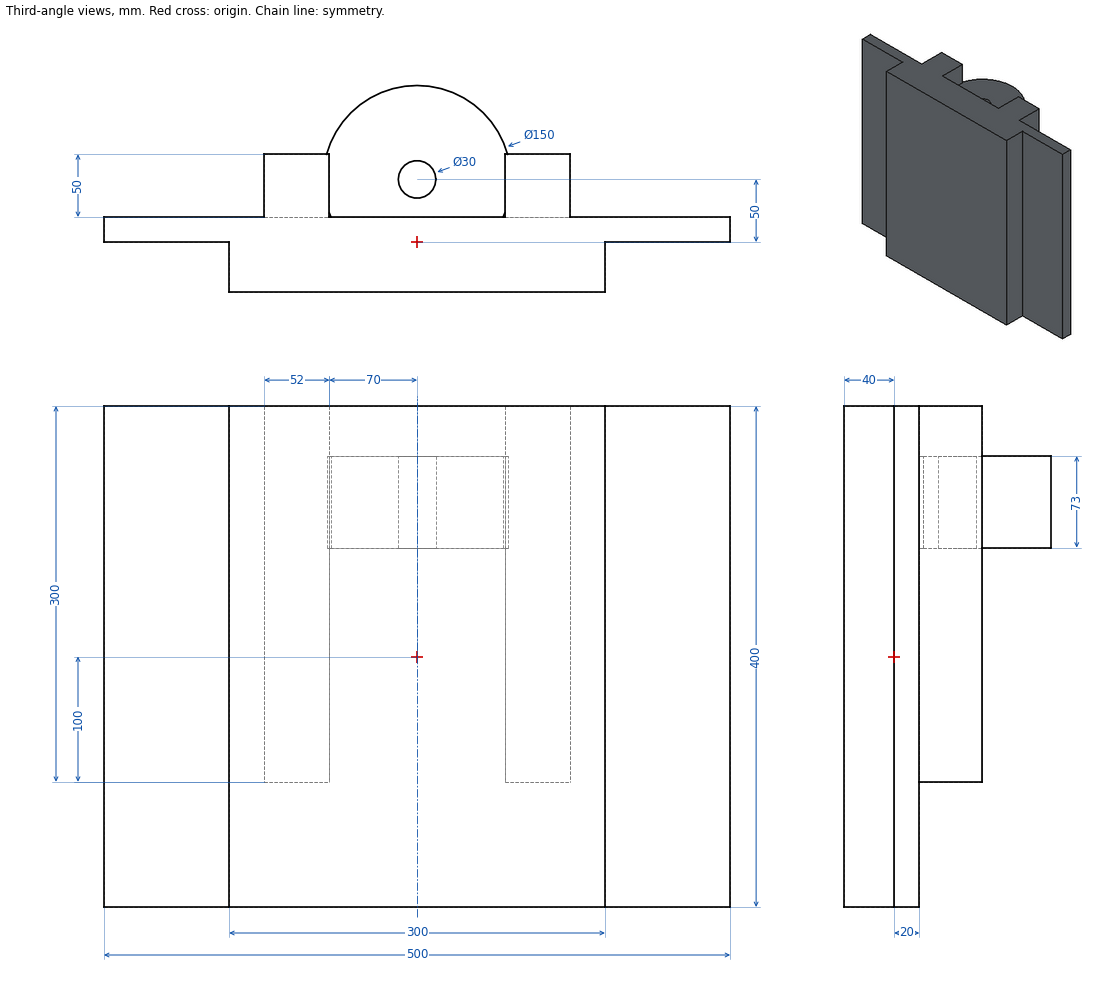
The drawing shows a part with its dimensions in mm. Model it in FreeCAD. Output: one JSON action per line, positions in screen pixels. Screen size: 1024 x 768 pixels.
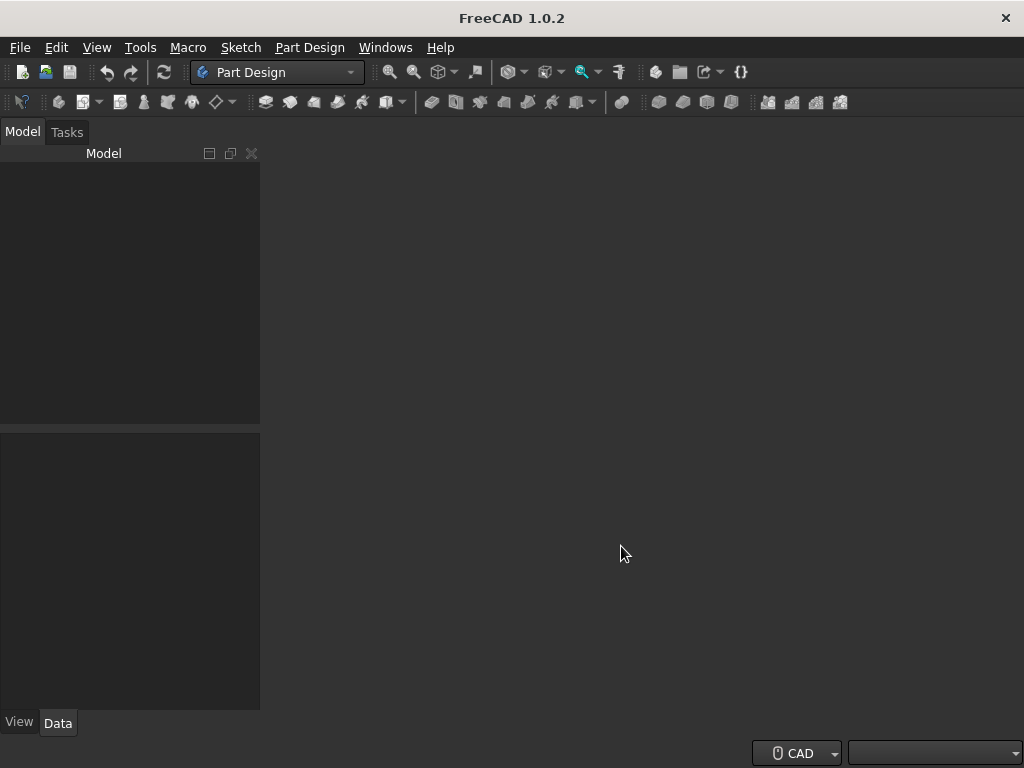
{"action": "key", "text": "ctrl+n"}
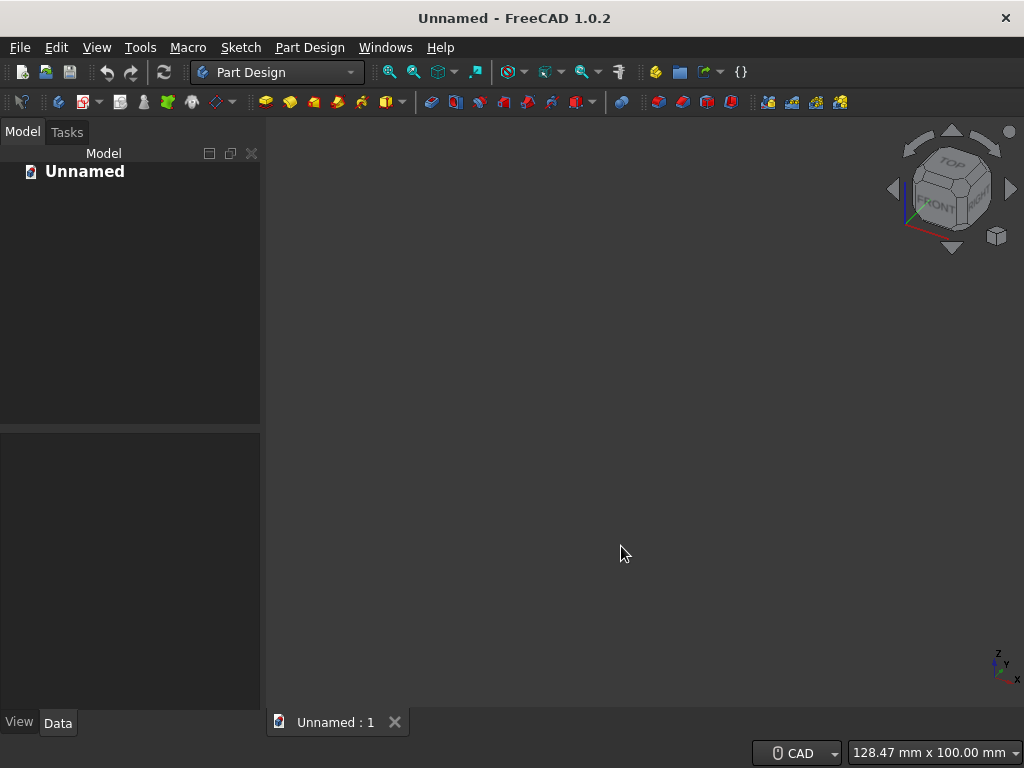
{"action": "left_click", "coordinate": [84, 102]}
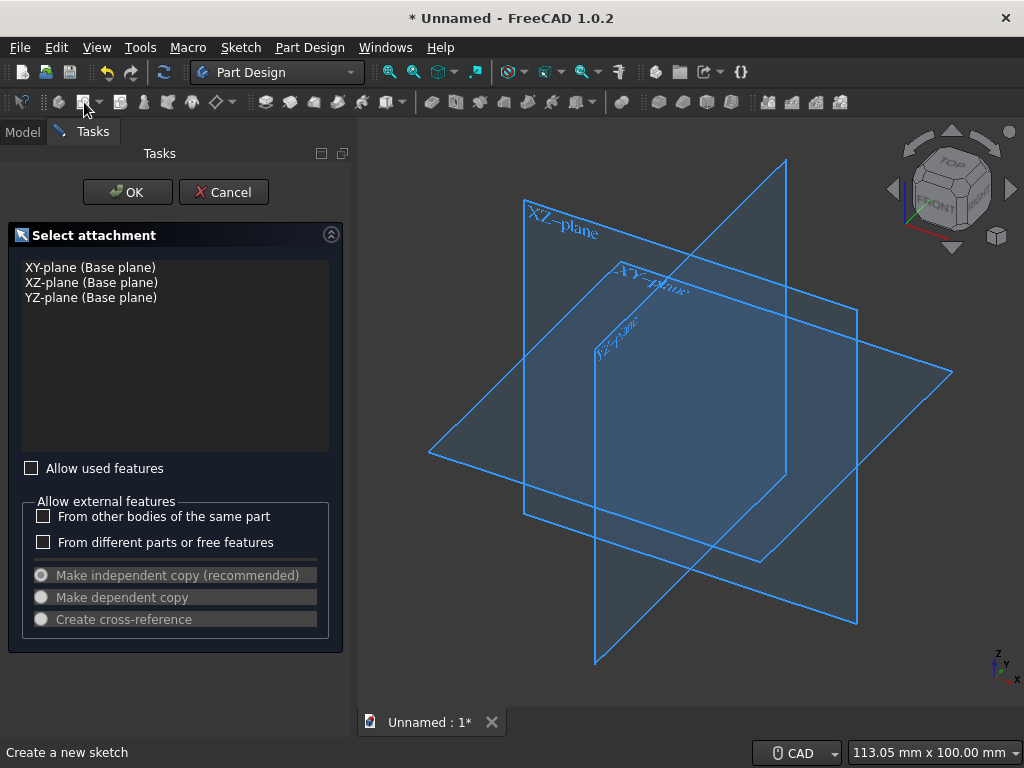
{"action": "left_click", "coordinate": [82, 282]}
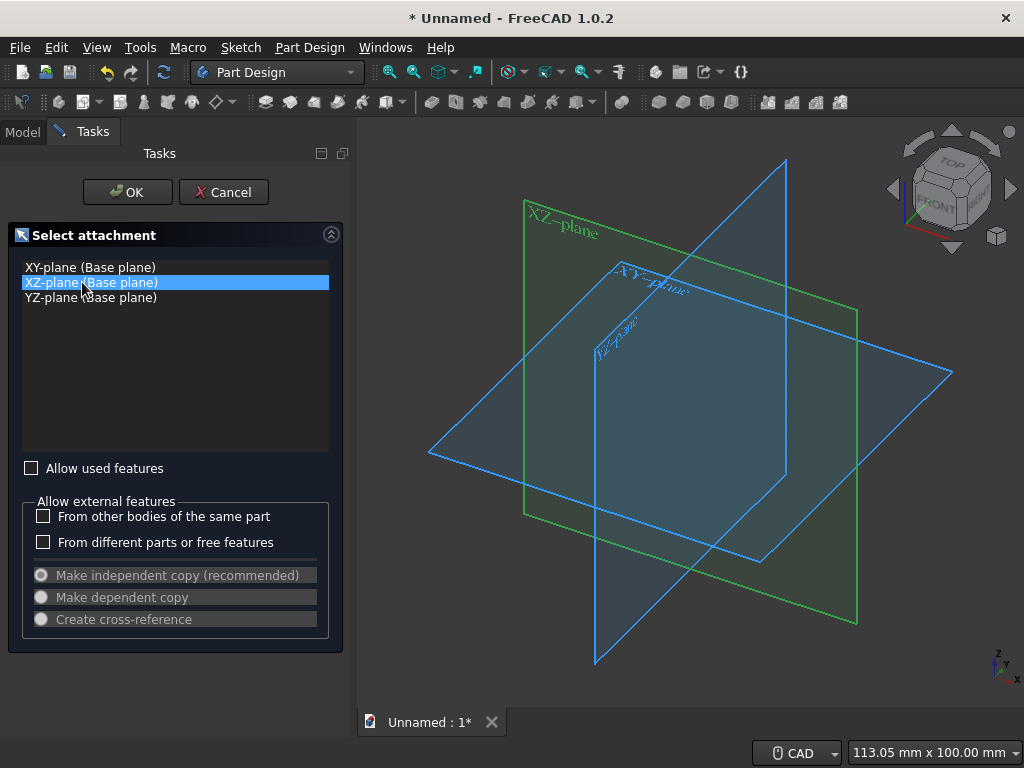
{"action": "left_click", "coordinate": [128, 192]}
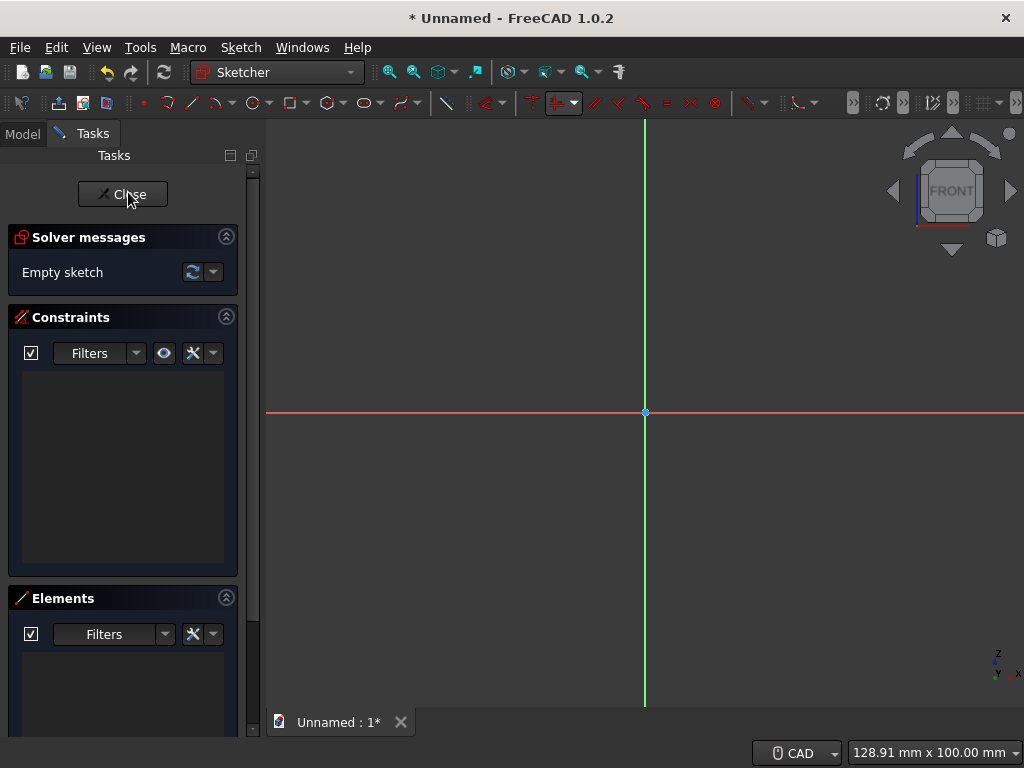
{"action": "scroll", "coordinate": [566, 413], "scroll_direction": "down", "scroll_amount": 10}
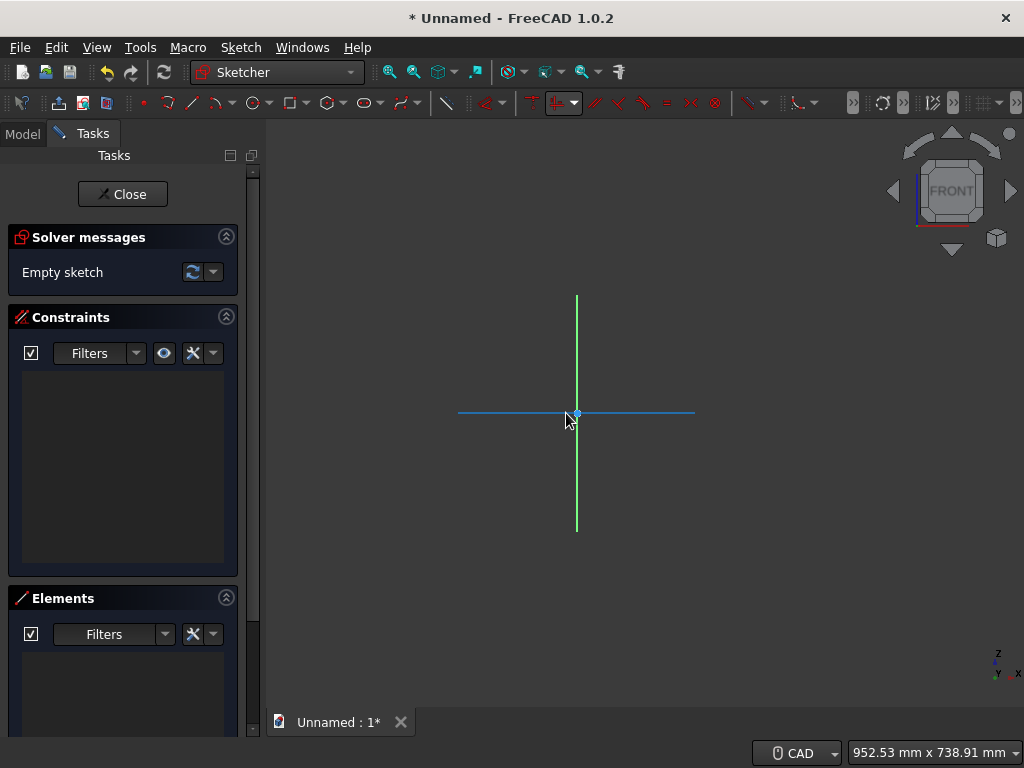
{"action": "left_click", "coordinate": [308, 104]}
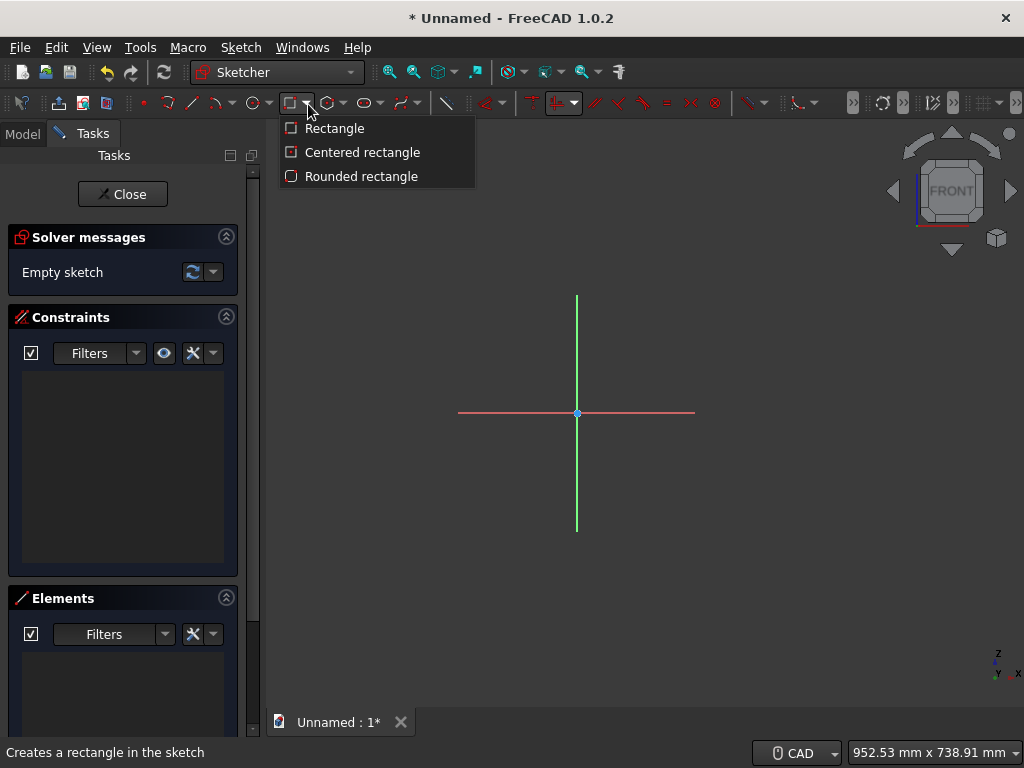
{"action": "left_click", "coordinate": [378, 152]}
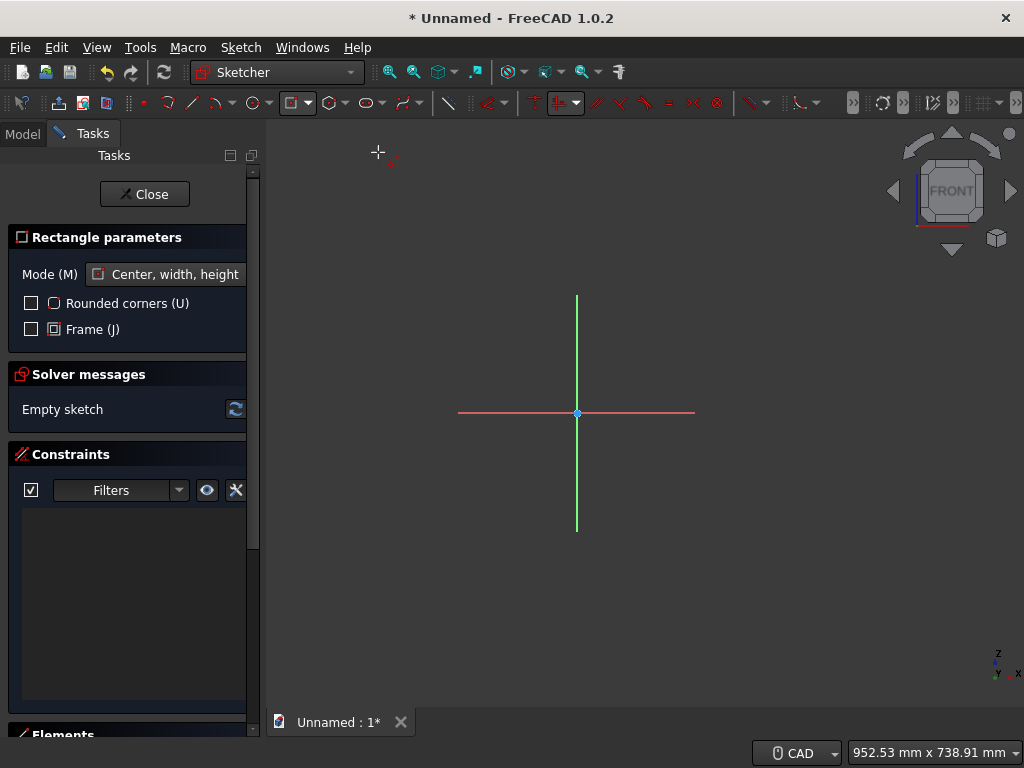
{"action": "left_click", "coordinate": [577, 413]}
{"action": "left_click", "coordinate": [776, 254]}
{"action": "key", "text": "Escape"}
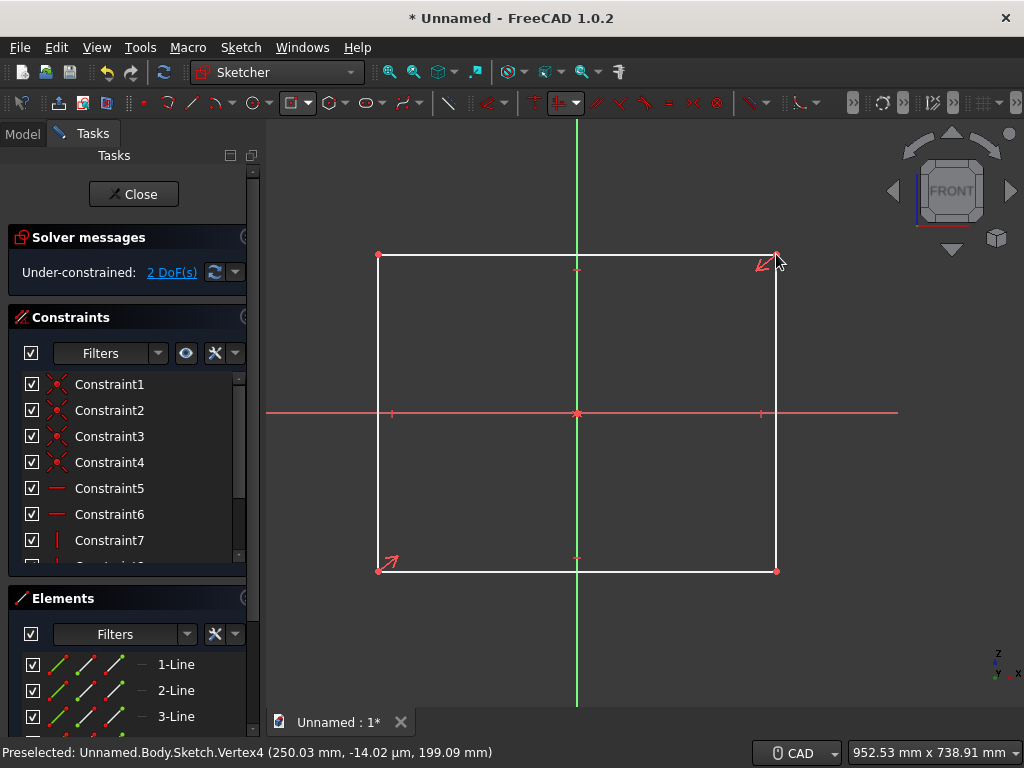
{"action": "left_click", "coordinate": [488, 104]}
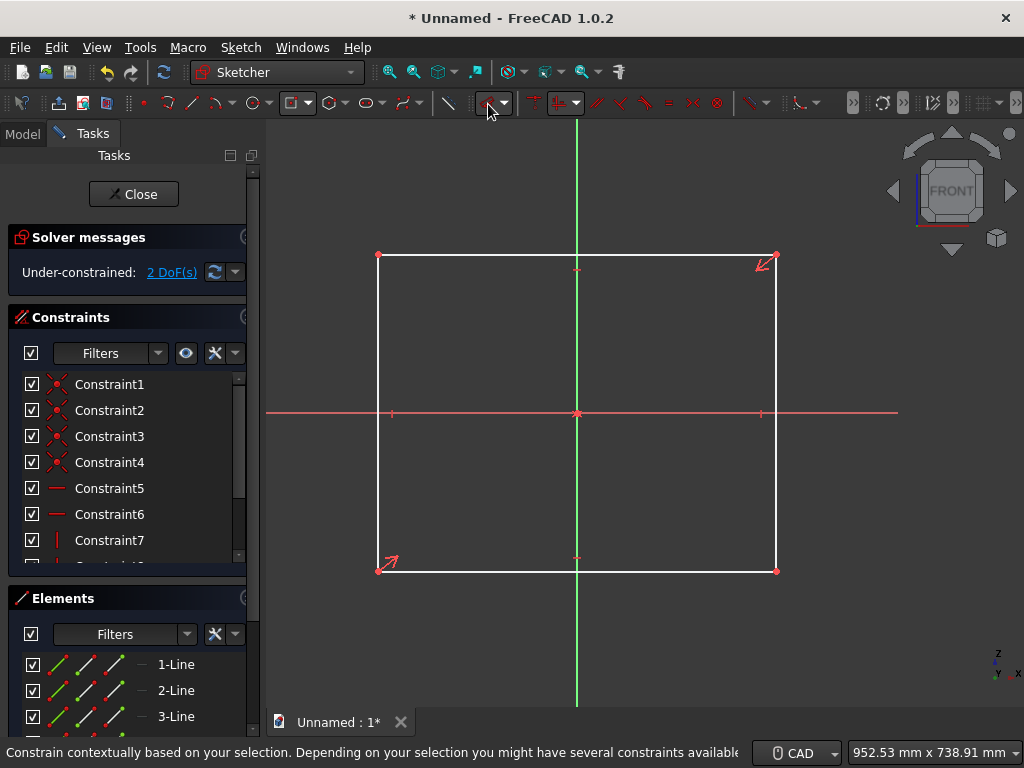
{"action": "left_click", "coordinate": [497, 572]}
{"action": "left_click", "coordinate": [486, 606]}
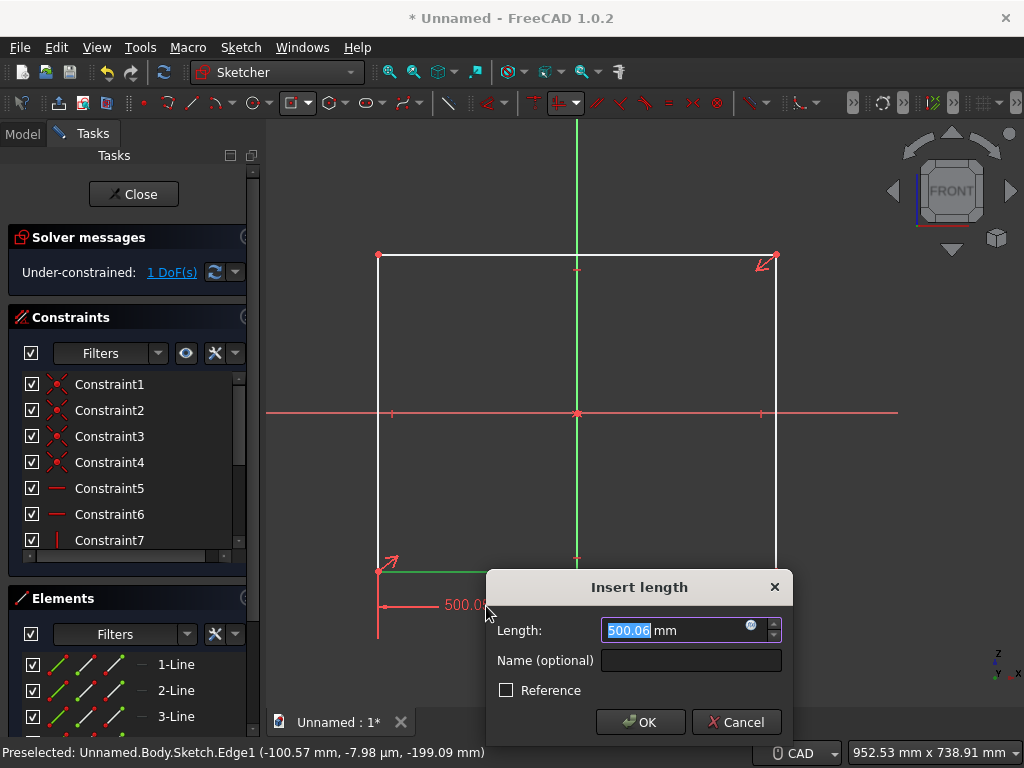
{"action": "type", "text": "500"}
{"action": "key", "text": "Return"}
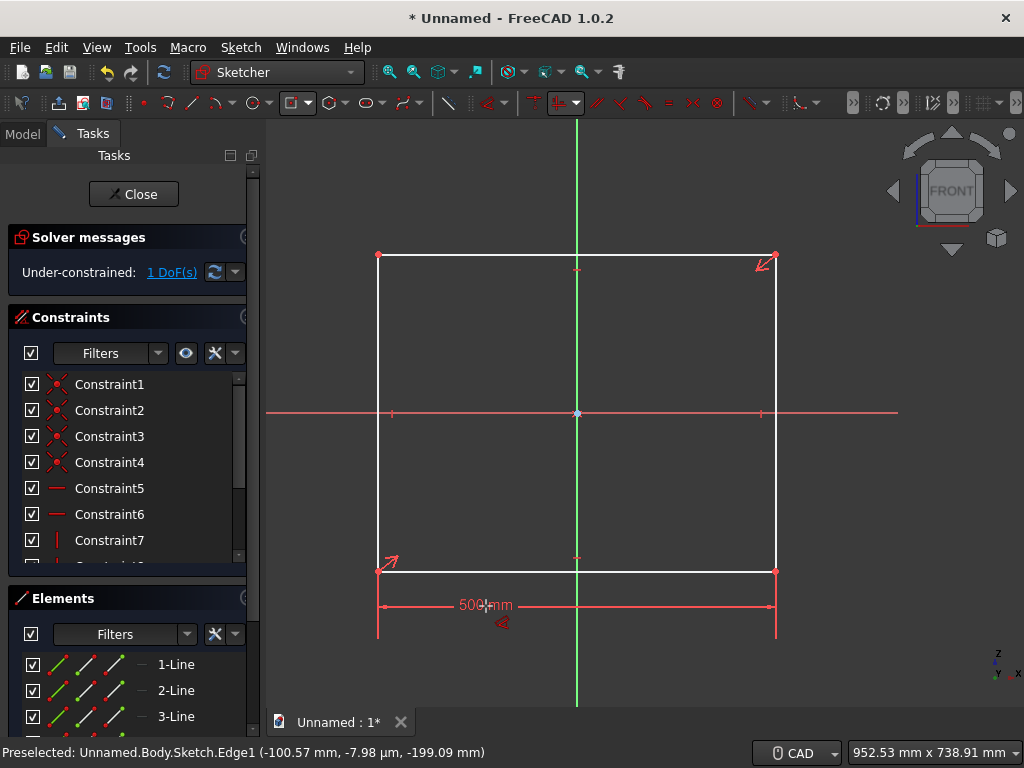
{"action": "left_click", "coordinate": [776, 477]}
{"action": "left_click", "coordinate": [810, 341]}